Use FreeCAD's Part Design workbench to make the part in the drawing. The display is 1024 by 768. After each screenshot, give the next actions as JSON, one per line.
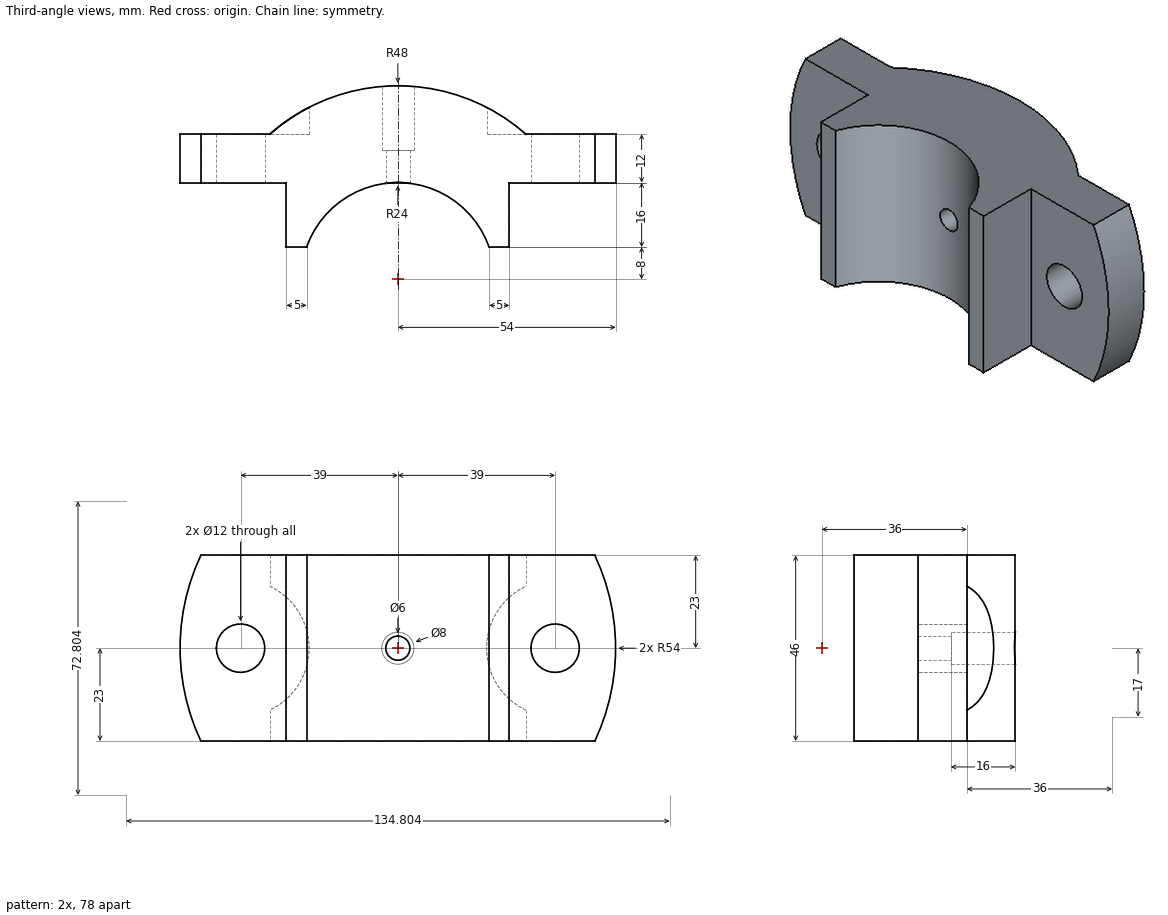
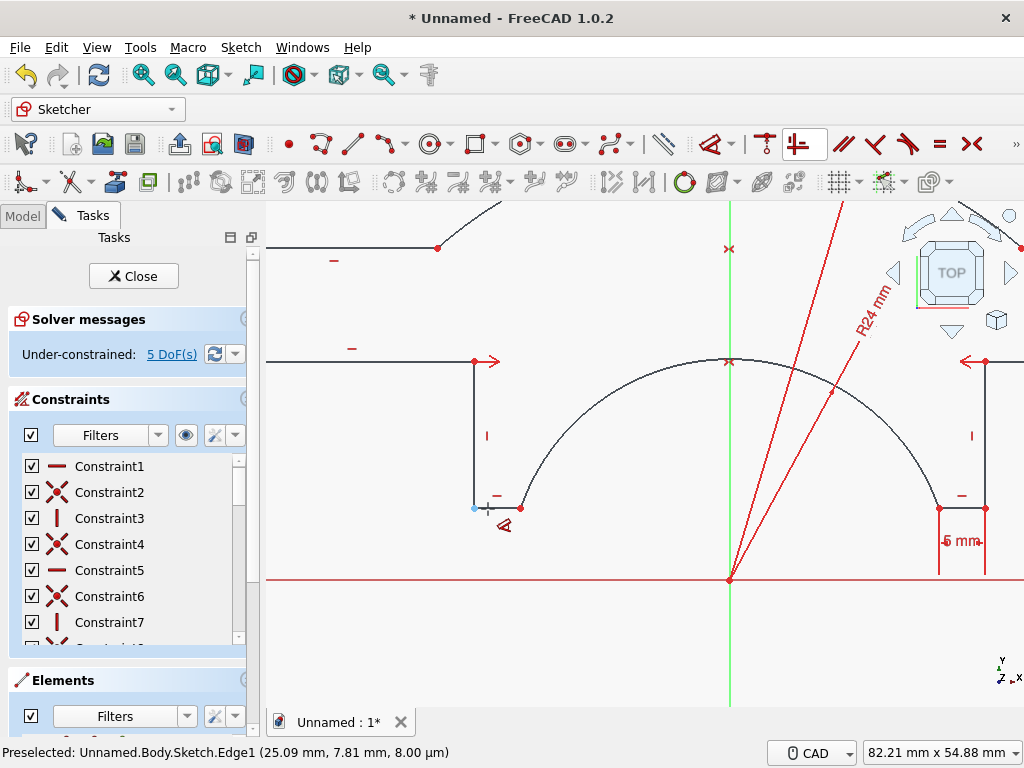
{"action": "left_click", "coordinate": [488, 508]}
{"action": "left_click", "coordinate": [498, 542]}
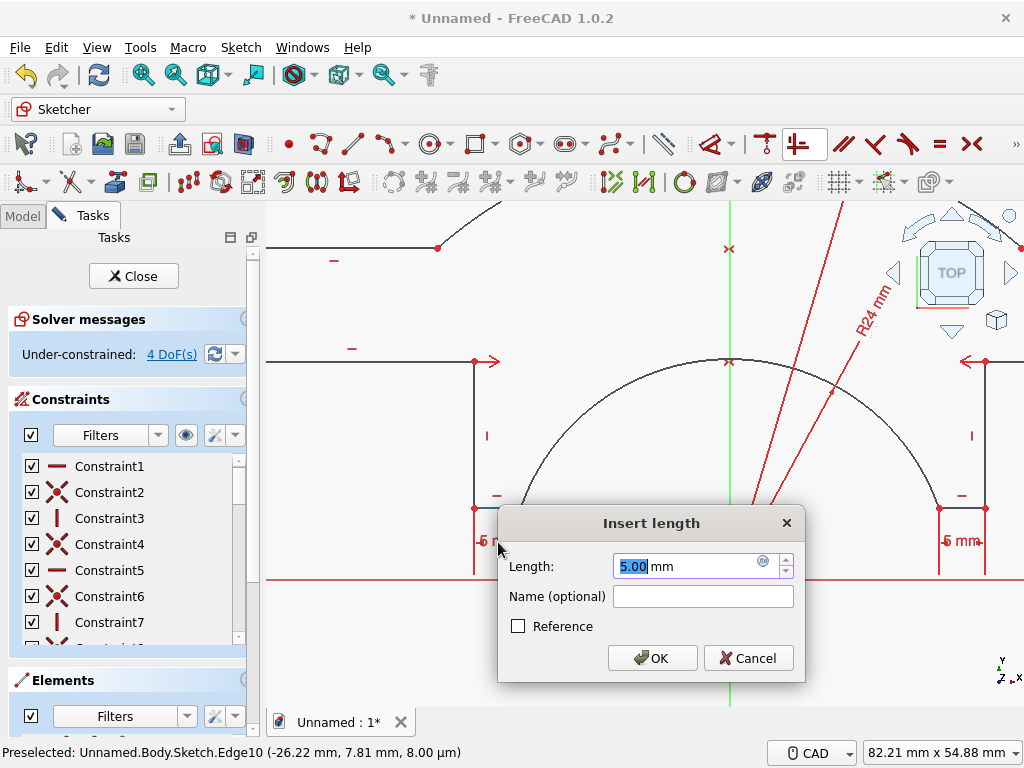
{"action": "type", "text": "5"}
{"action": "key", "text": "Return"}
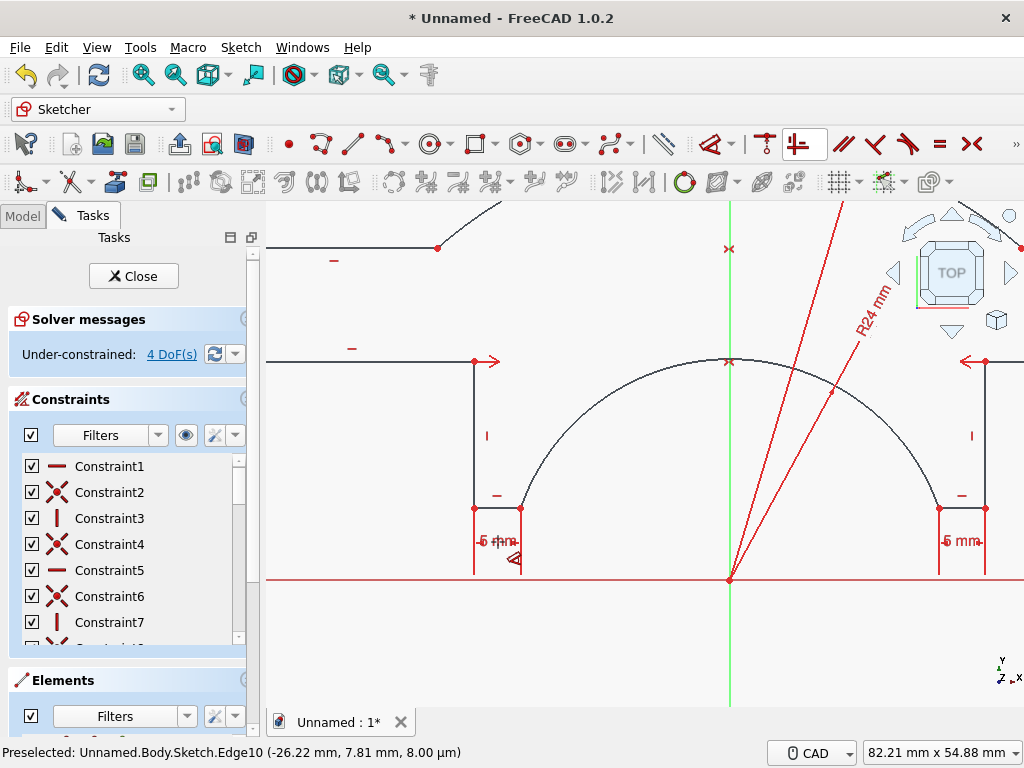
{"action": "scroll", "coordinate": [487, 509], "scroll_direction": "down", "scroll_amount": 5}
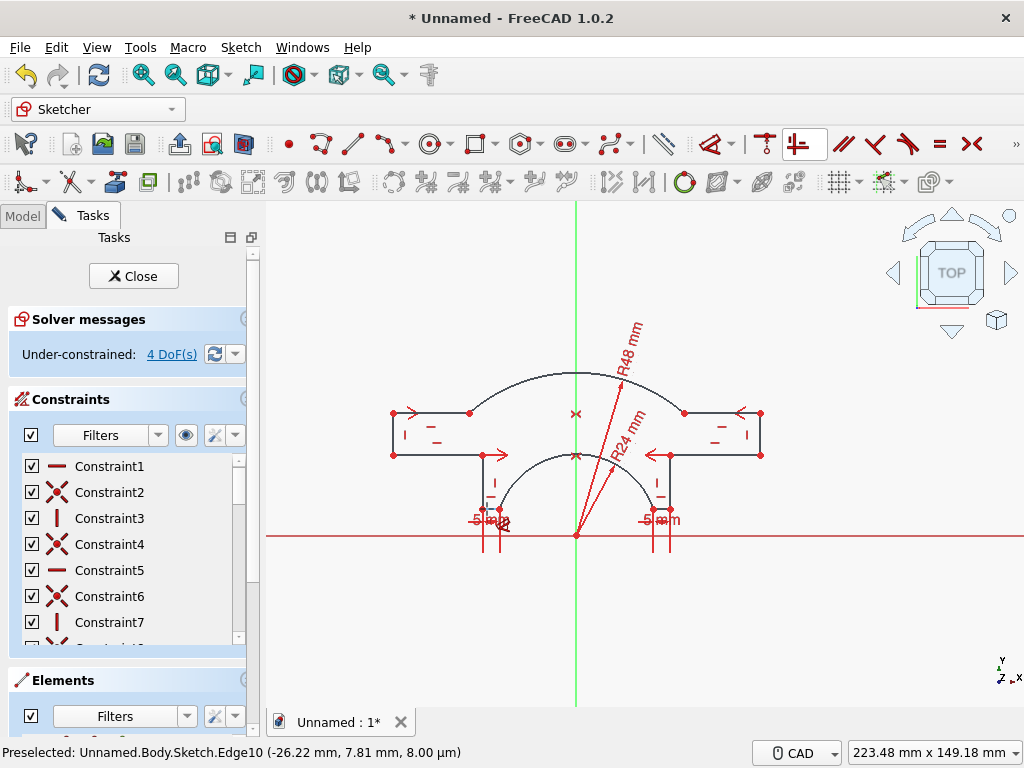
{"action": "left_click", "coordinate": [670, 493]}
{"action": "left_click", "coordinate": [704, 482]}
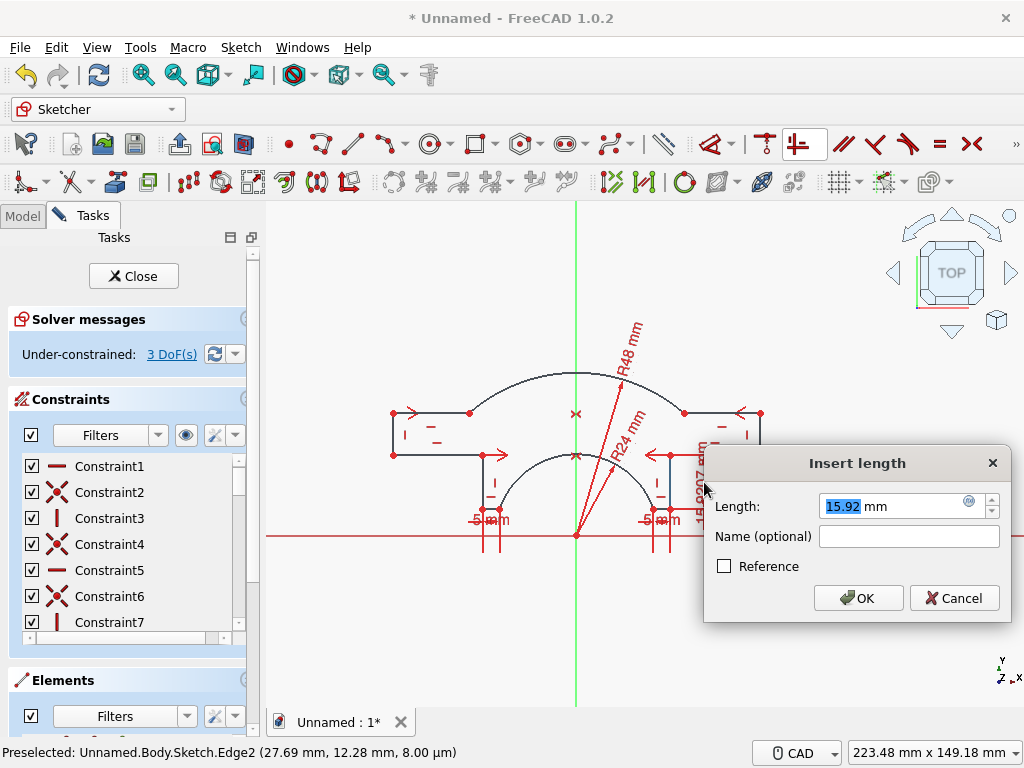
{"action": "type", "text": "16"}
{"action": "key", "text": "Return"}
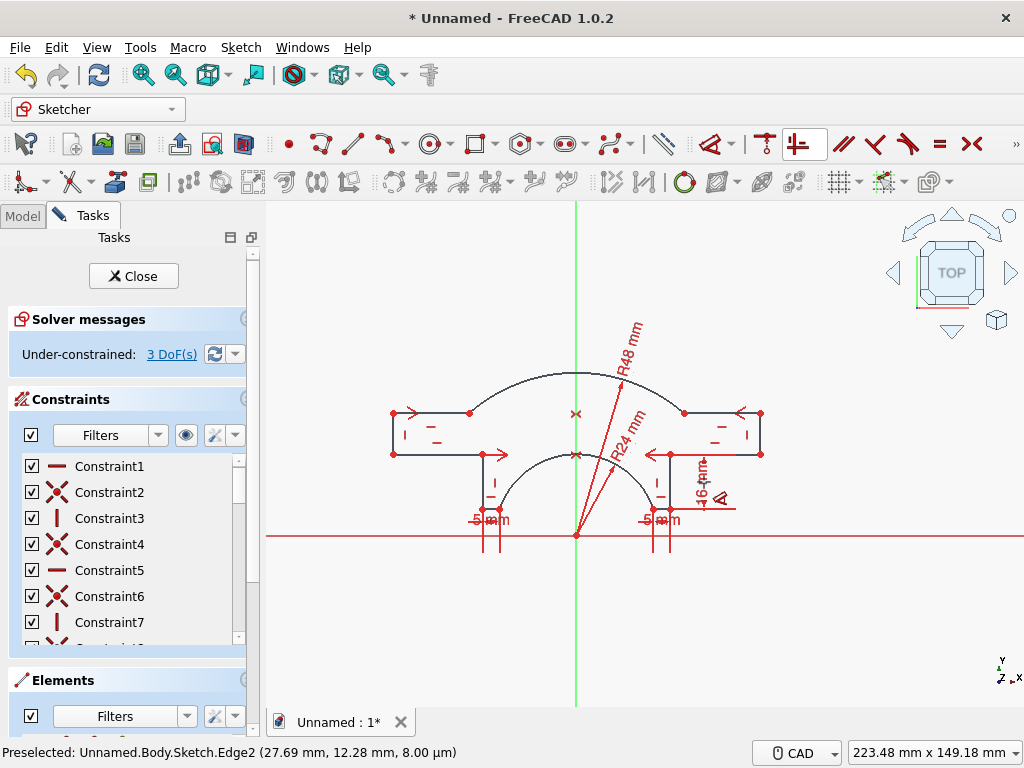
{"action": "left_click", "coordinate": [760, 442]}
{"action": "left_click", "coordinate": [794, 434]}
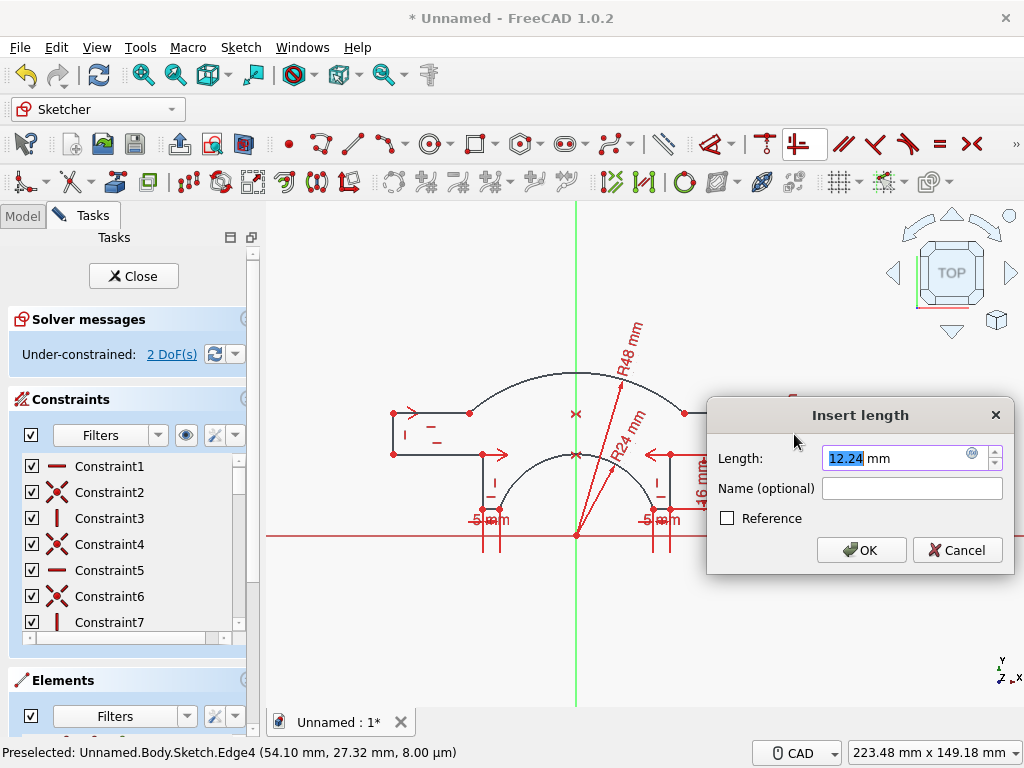
{"action": "type", "text": "12"}
{"action": "key", "text": "Return"}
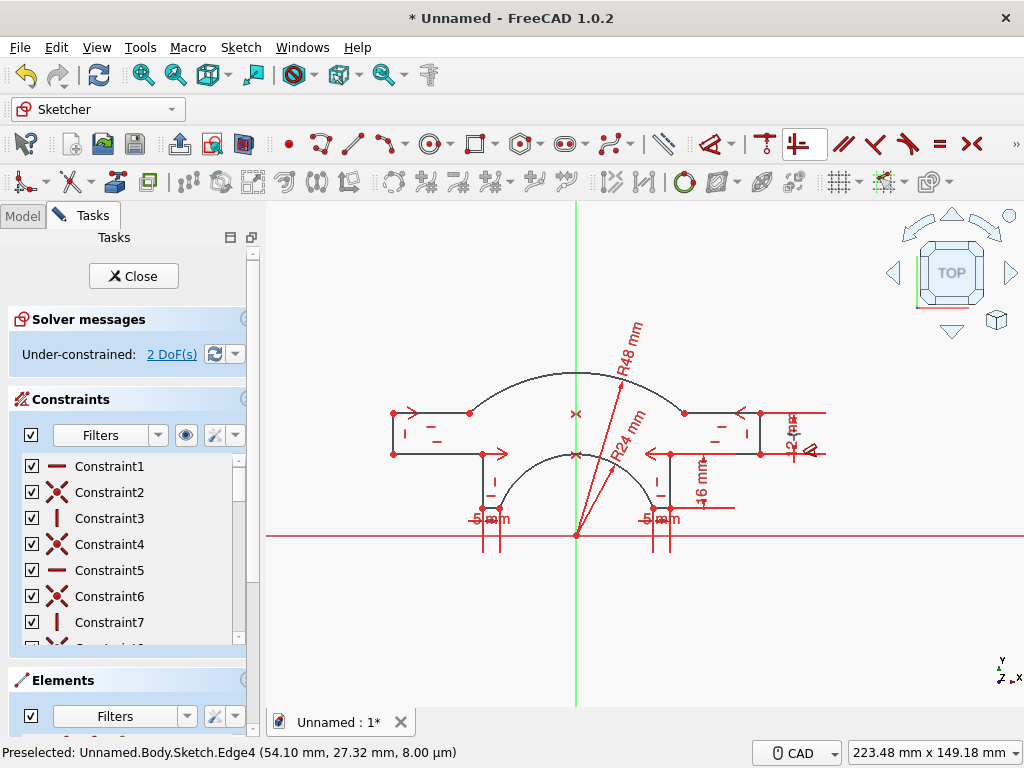
{"action": "scroll", "coordinate": [653, 508], "scroll_direction": "up", "scroll_amount": 2}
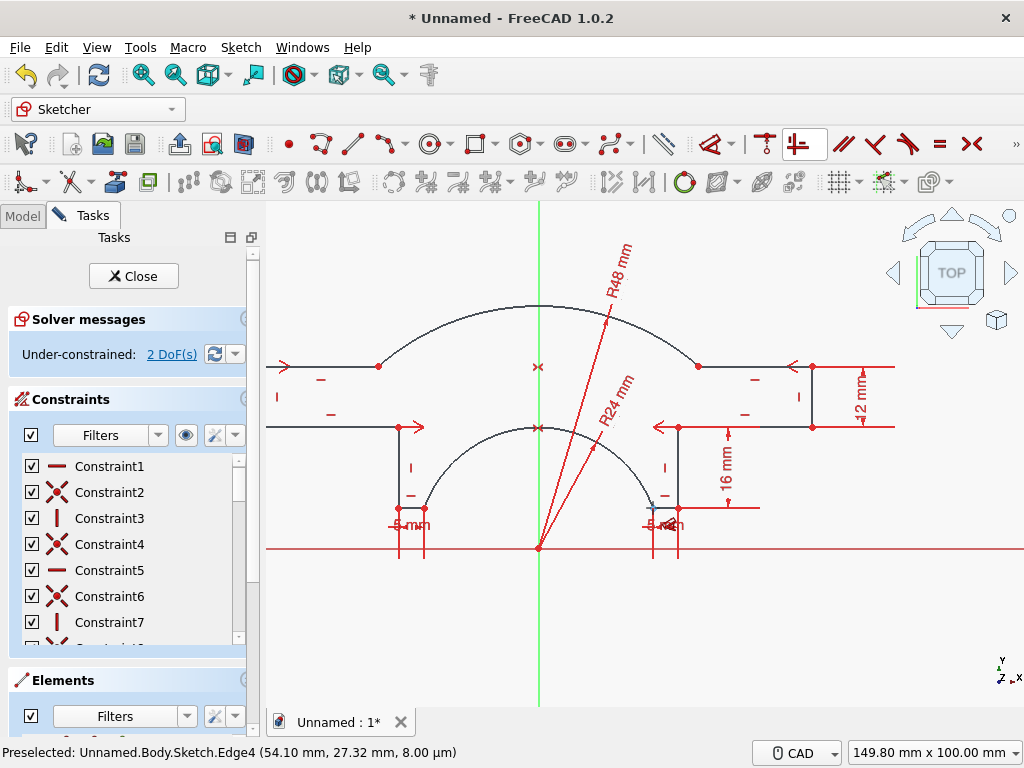
{"action": "left_click", "coordinate": [653, 508]}
{"action": "left_click", "coordinate": [505, 529]}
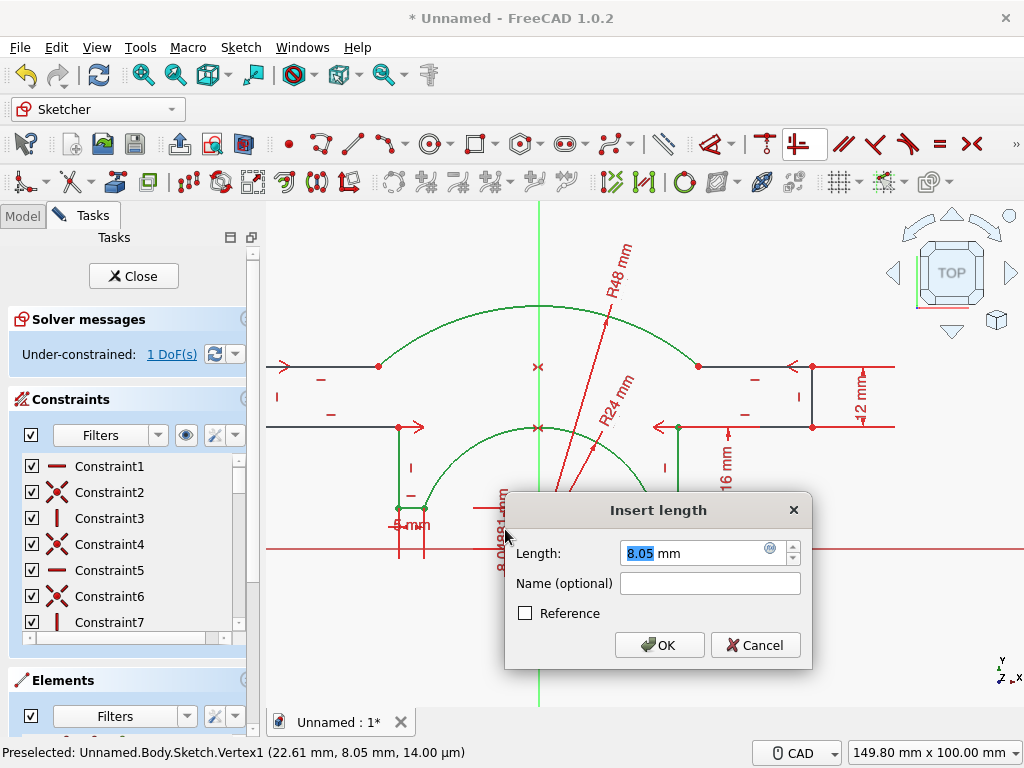
{"action": "type", "text": "8"}
{"action": "key", "text": "Return"}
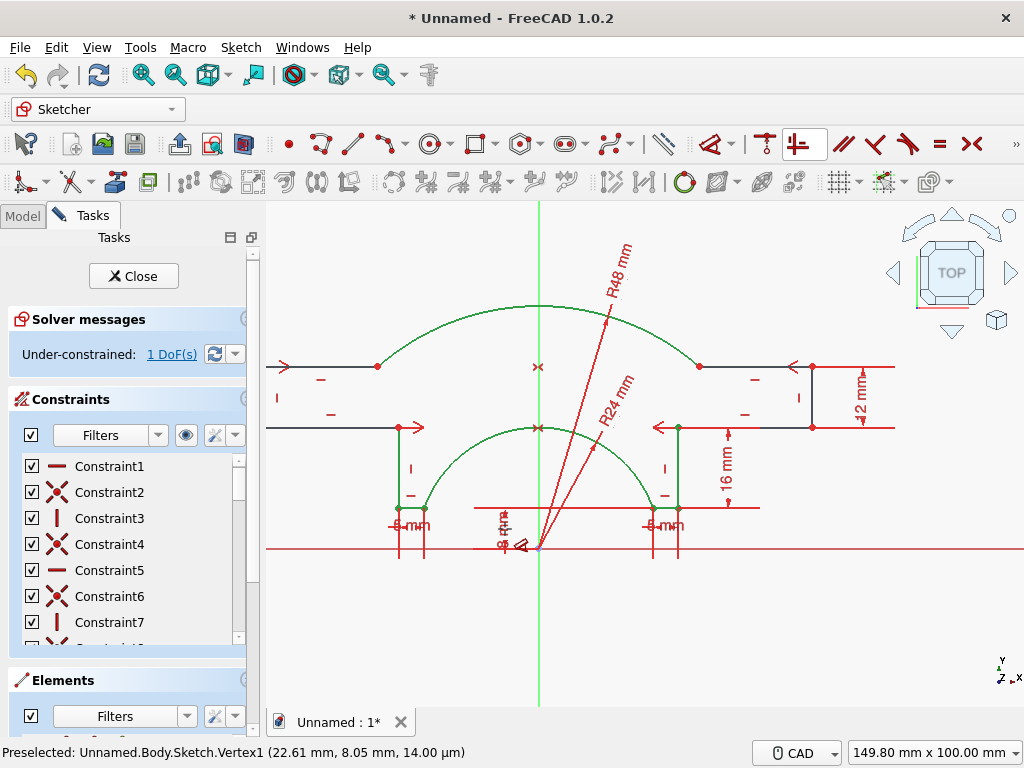
{"action": "left_click", "coordinate": [812, 428]}
{"action": "left_click", "coordinate": [675, 583]}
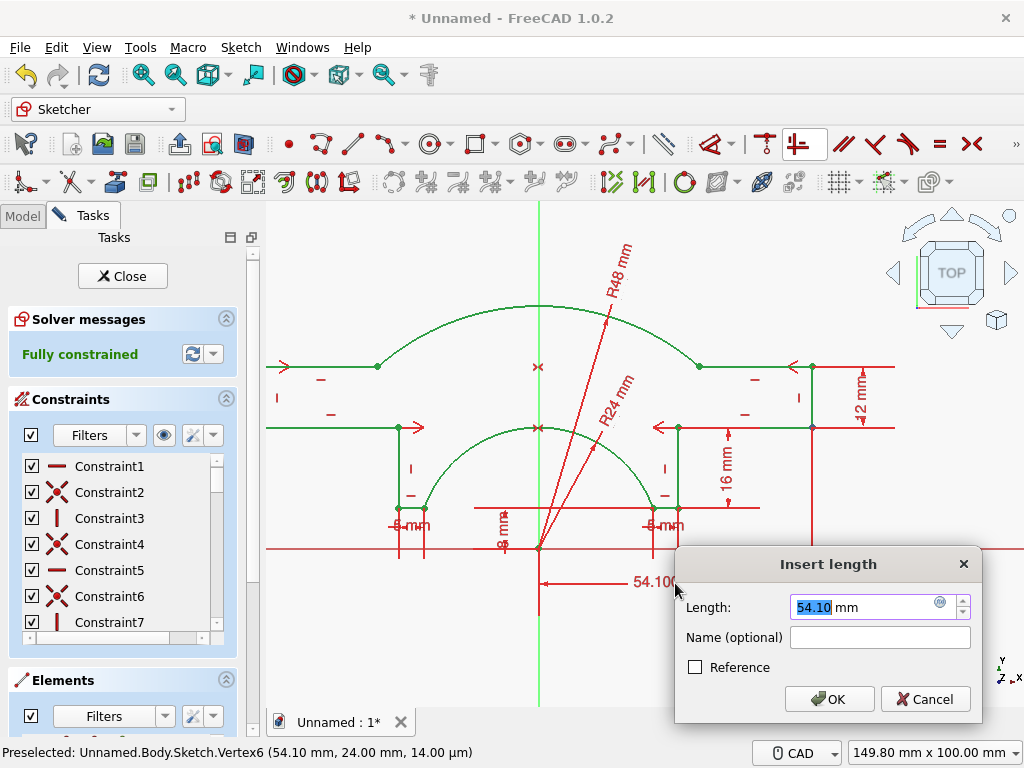
{"action": "type", "text": "54"}
{"action": "key", "text": "Return"}
{"action": "key", "text": "Escape"}